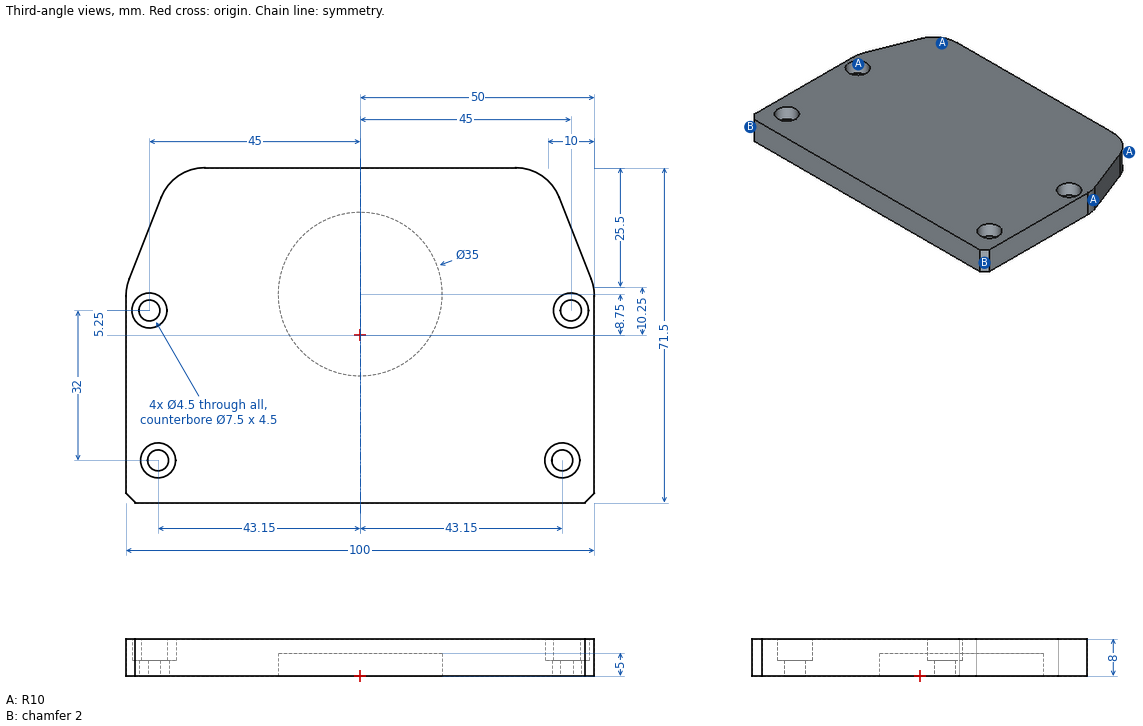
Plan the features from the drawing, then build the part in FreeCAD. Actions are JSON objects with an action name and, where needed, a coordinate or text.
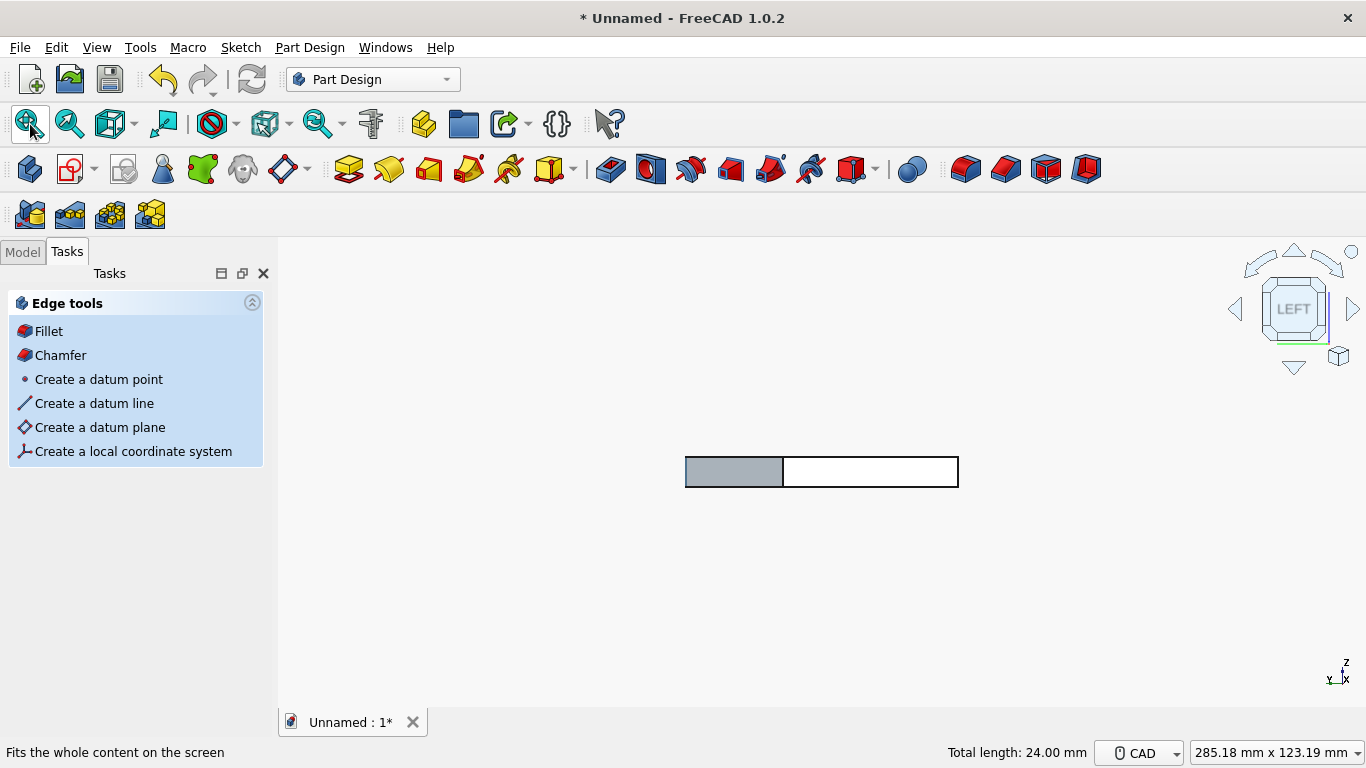
{"action": "left_click", "coordinate": [783, 471], "text": "ctrl"}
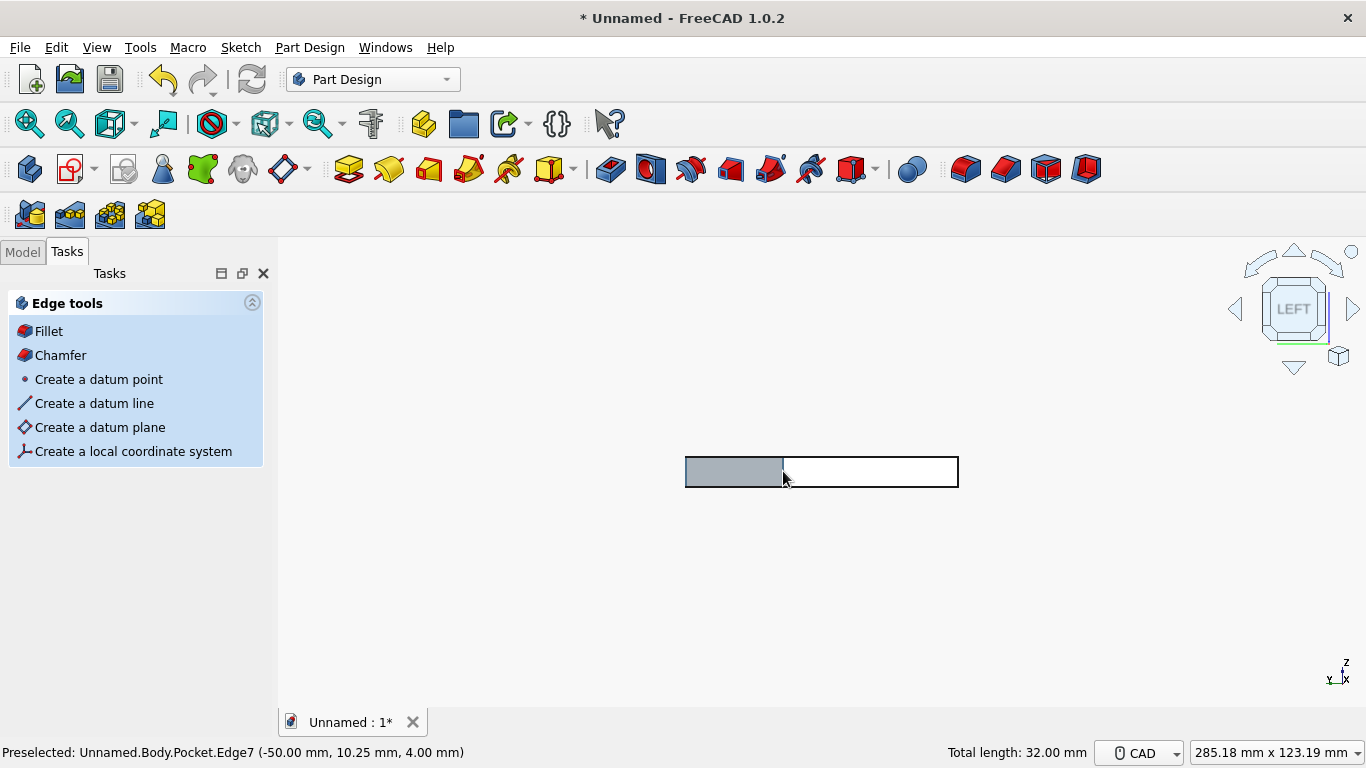
{"action": "left_click", "coordinate": [966, 170]}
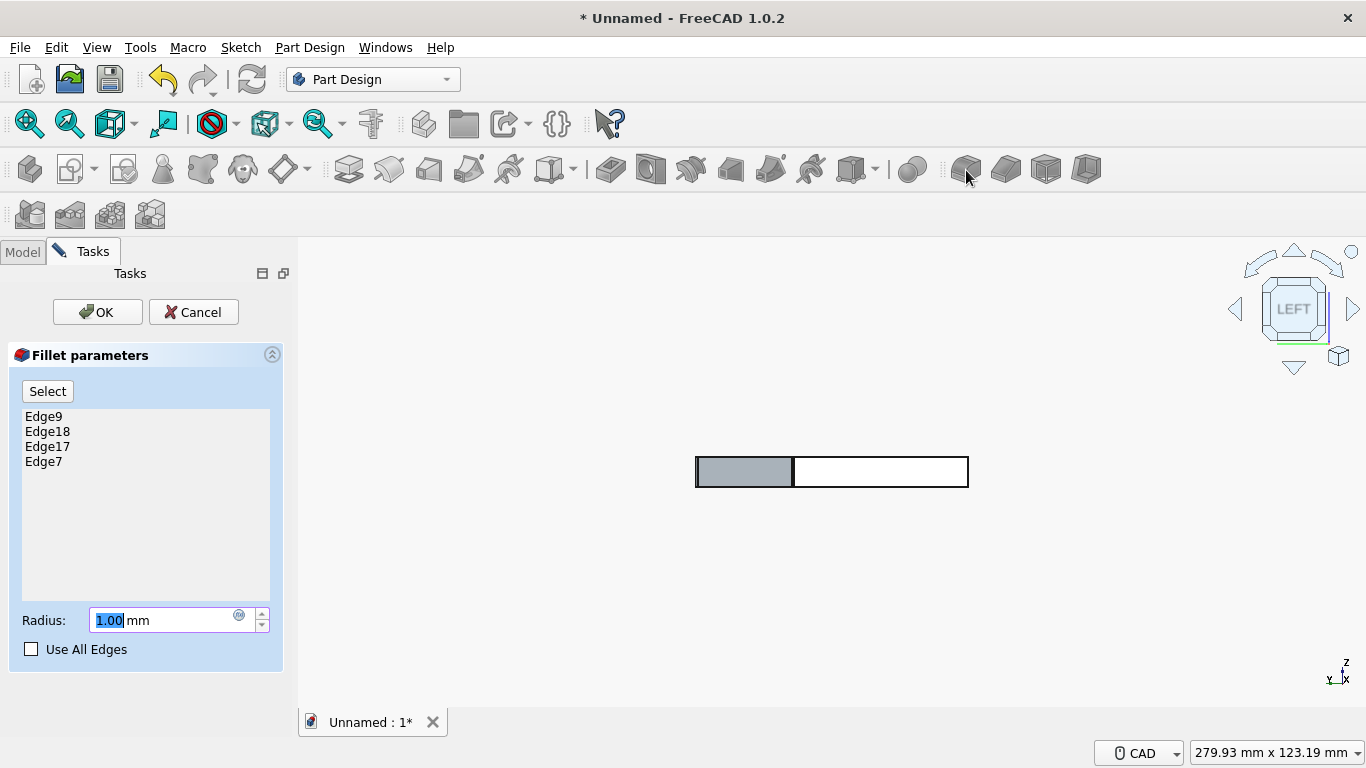
{"action": "type", "text": "10"}
{"action": "key", "text": "Tab"}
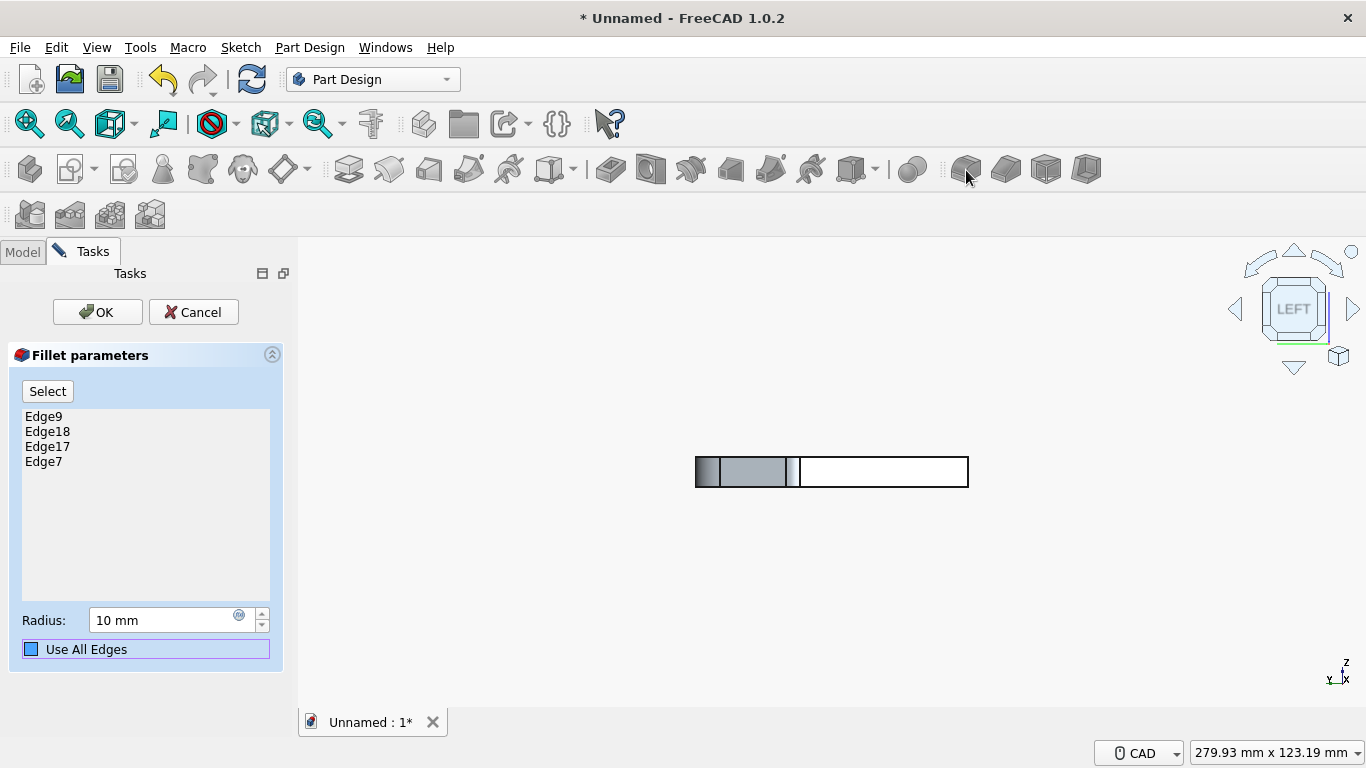
{"action": "left_click", "coordinate": [98, 312]}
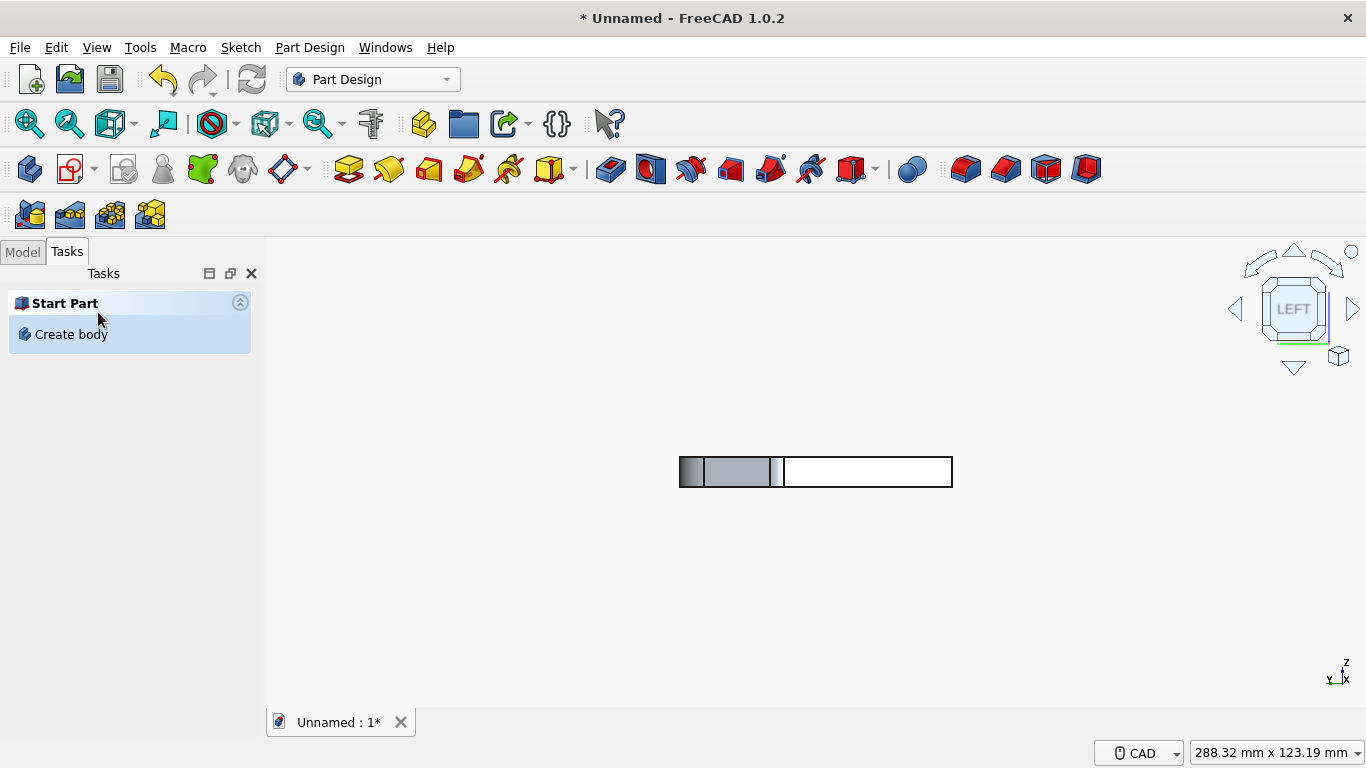
{"action": "left_click", "coordinate": [30, 124]}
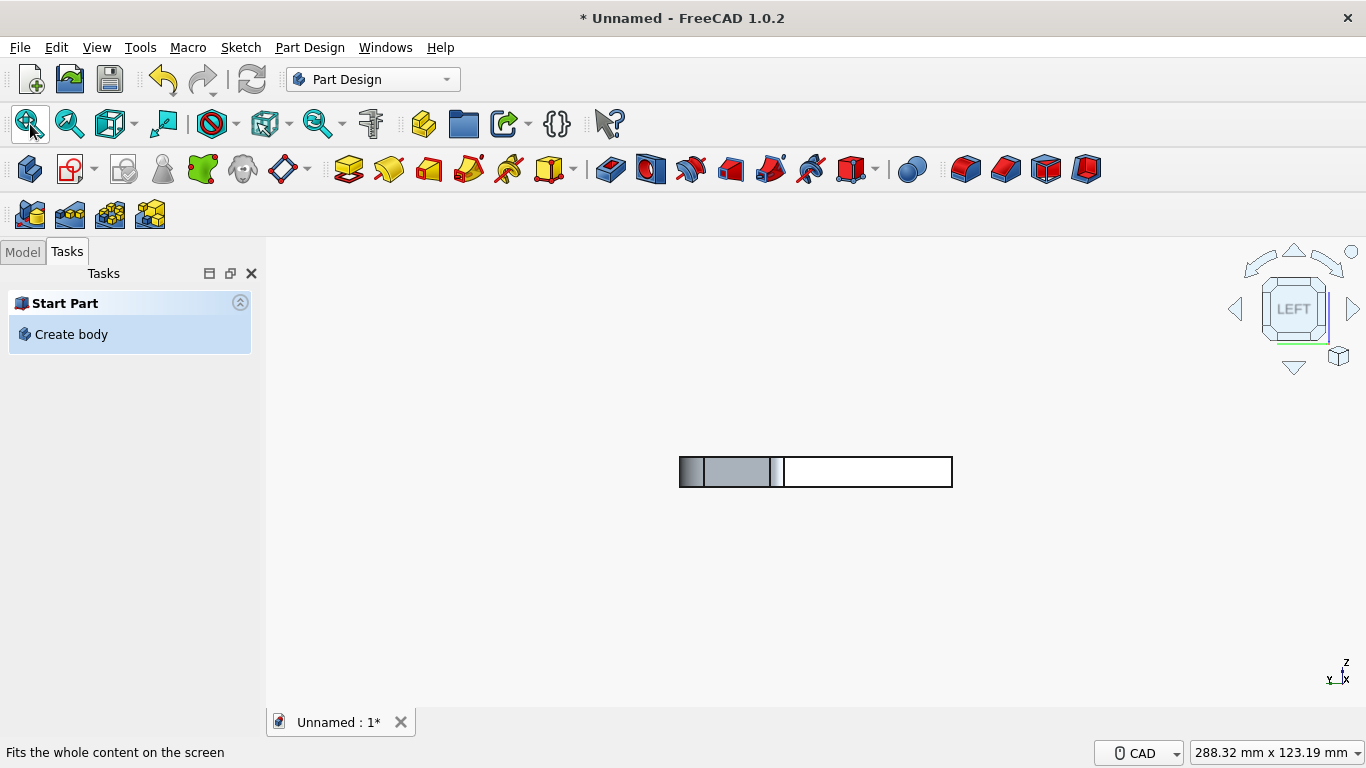
{"action": "left_click", "coordinate": [952, 471]}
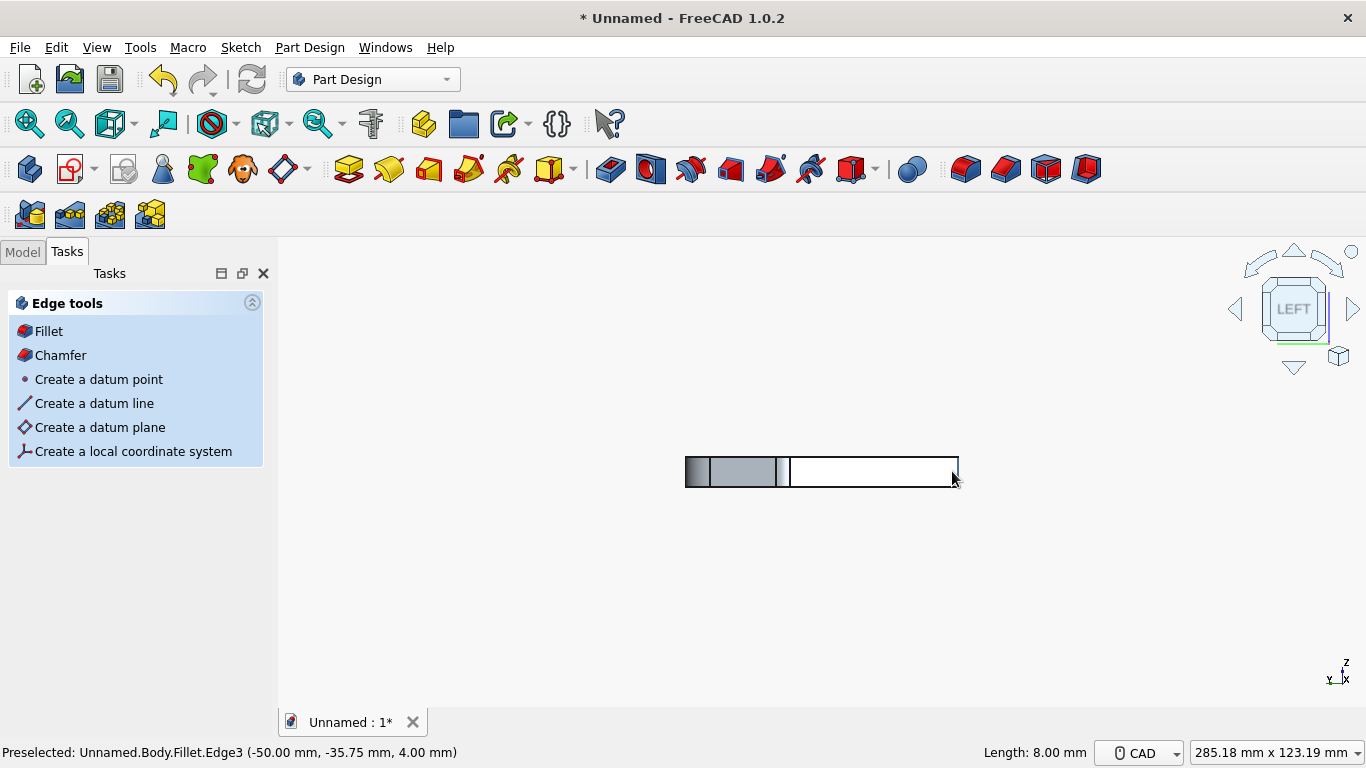
{"action": "key", "text": "0"}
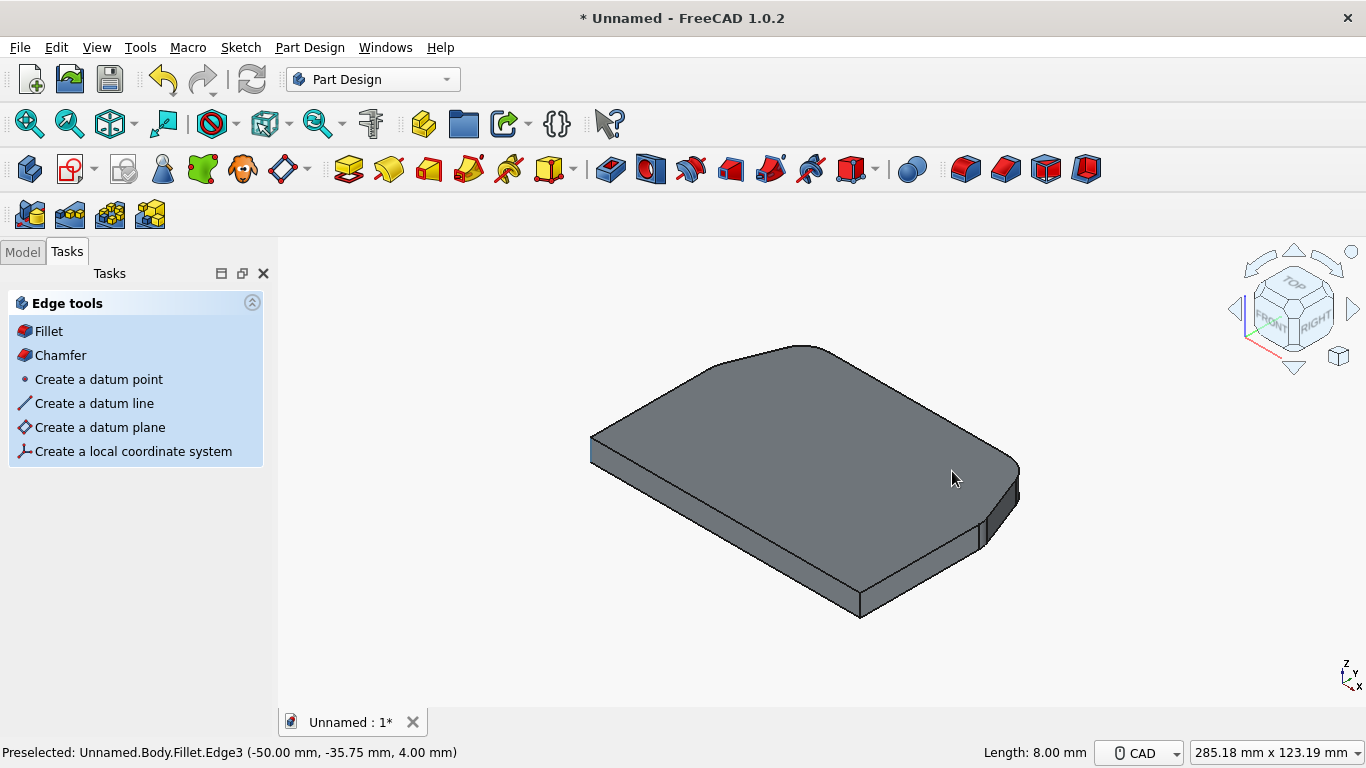
{"action": "left_click", "coordinate": [860, 605], "text": "ctrl"}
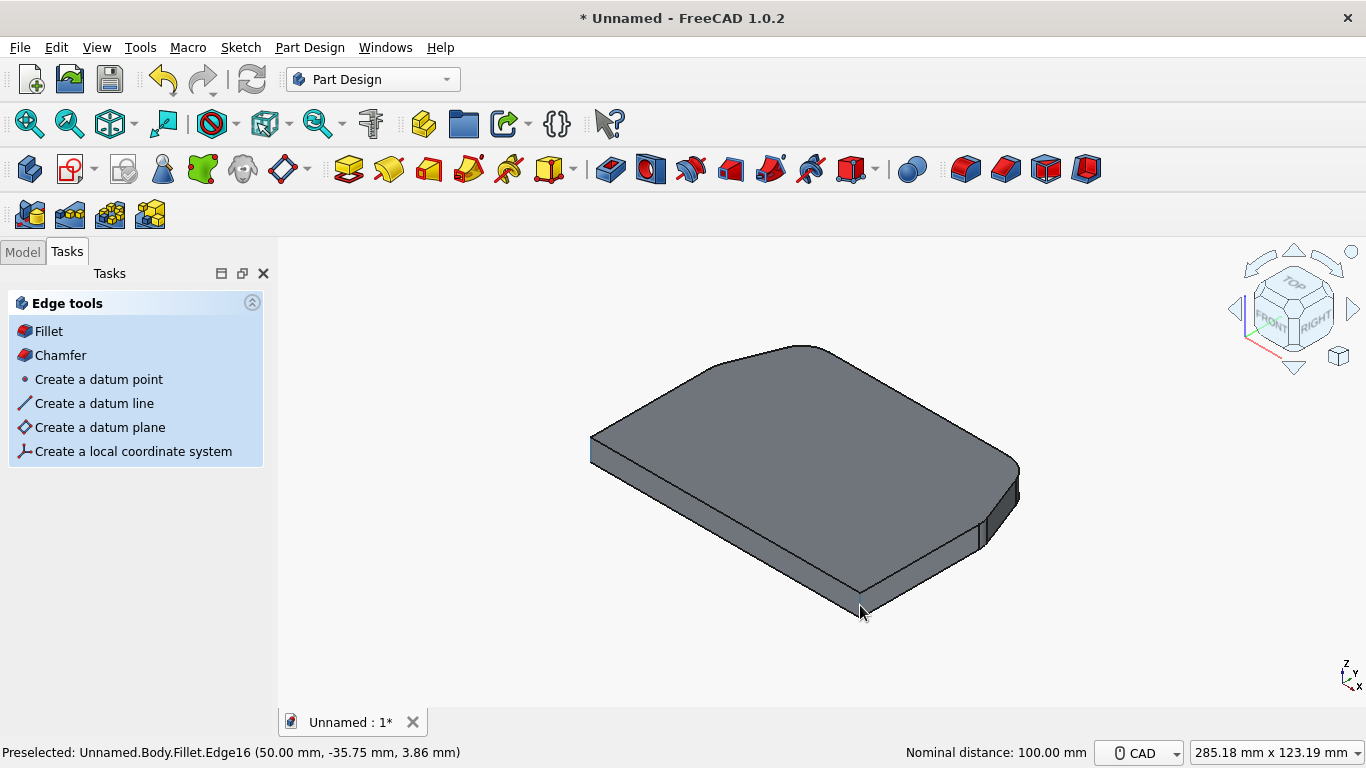
{"action": "left_click", "coordinate": [1006, 170]}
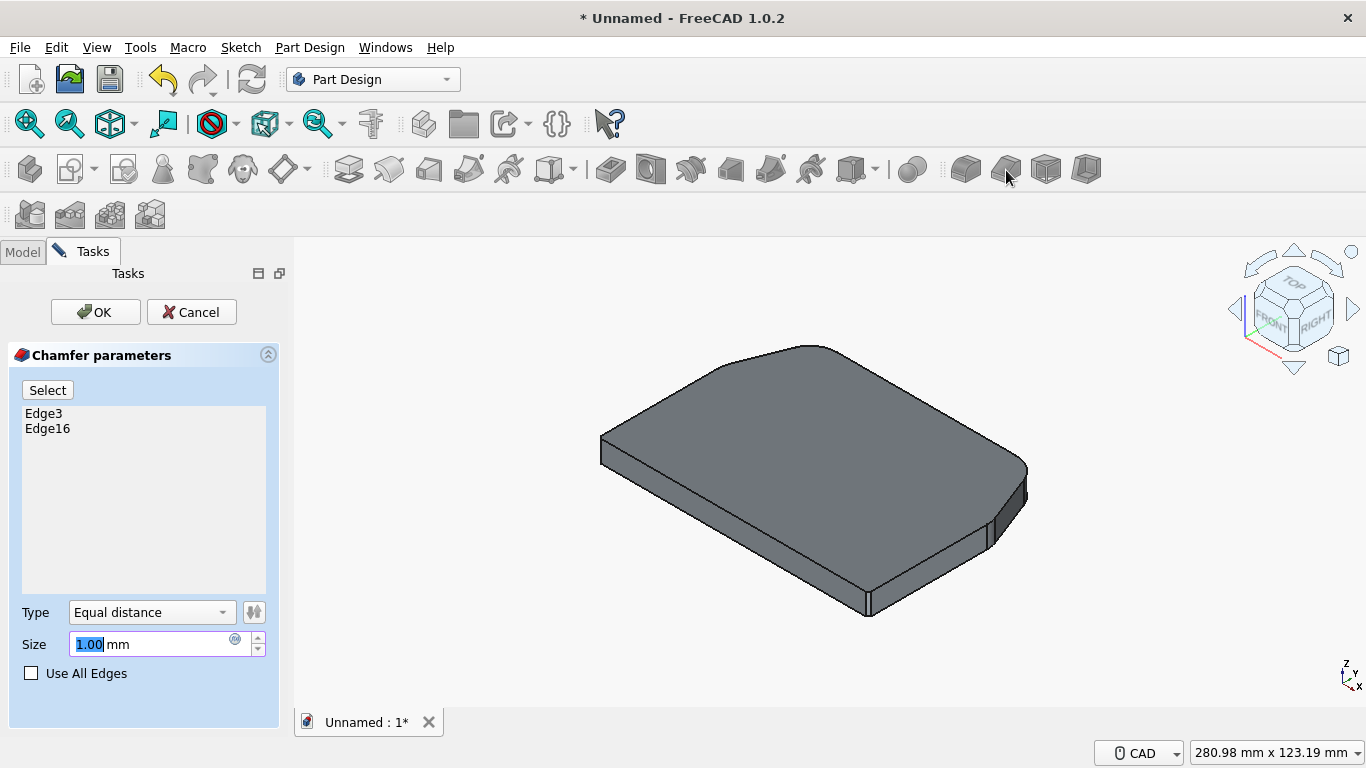
{"action": "type", "text": "2"}
{"action": "key", "text": "Tab"}